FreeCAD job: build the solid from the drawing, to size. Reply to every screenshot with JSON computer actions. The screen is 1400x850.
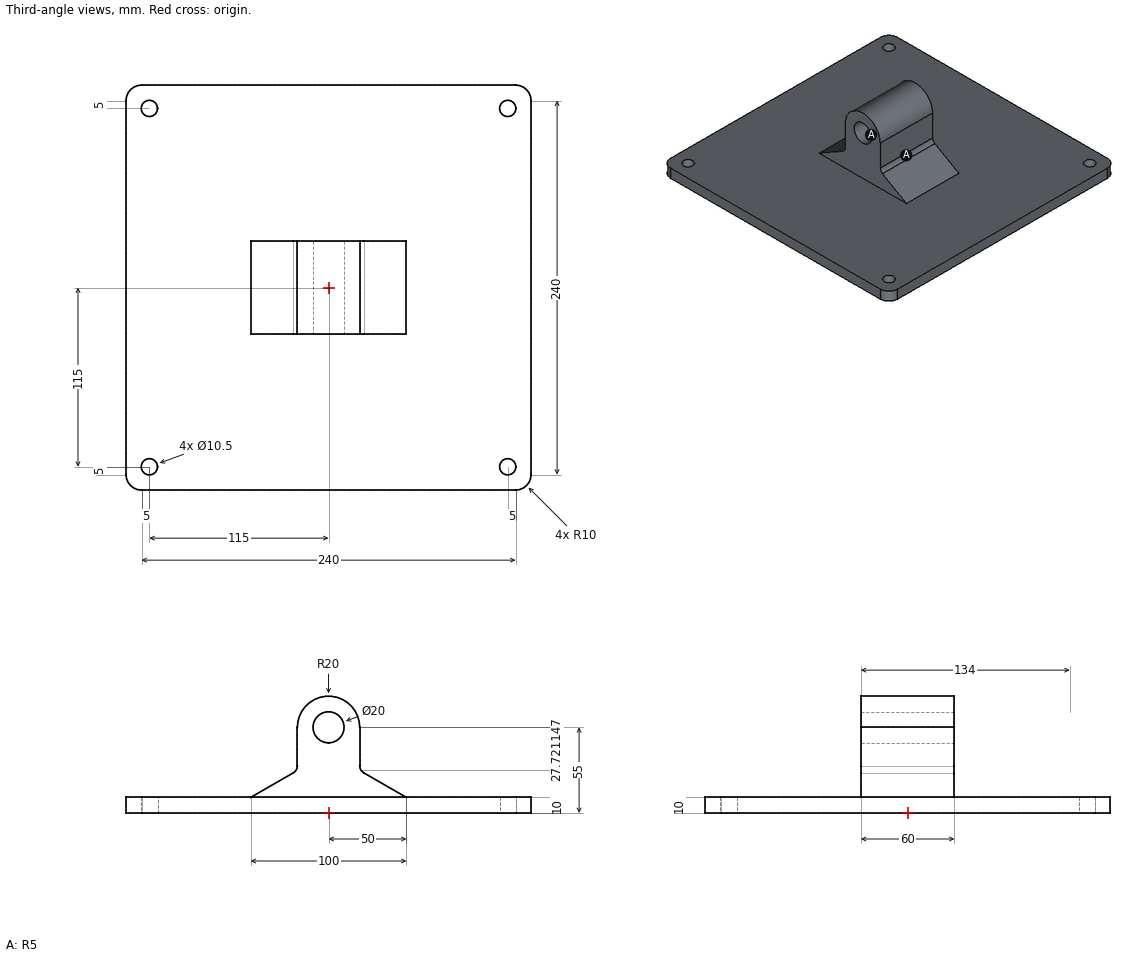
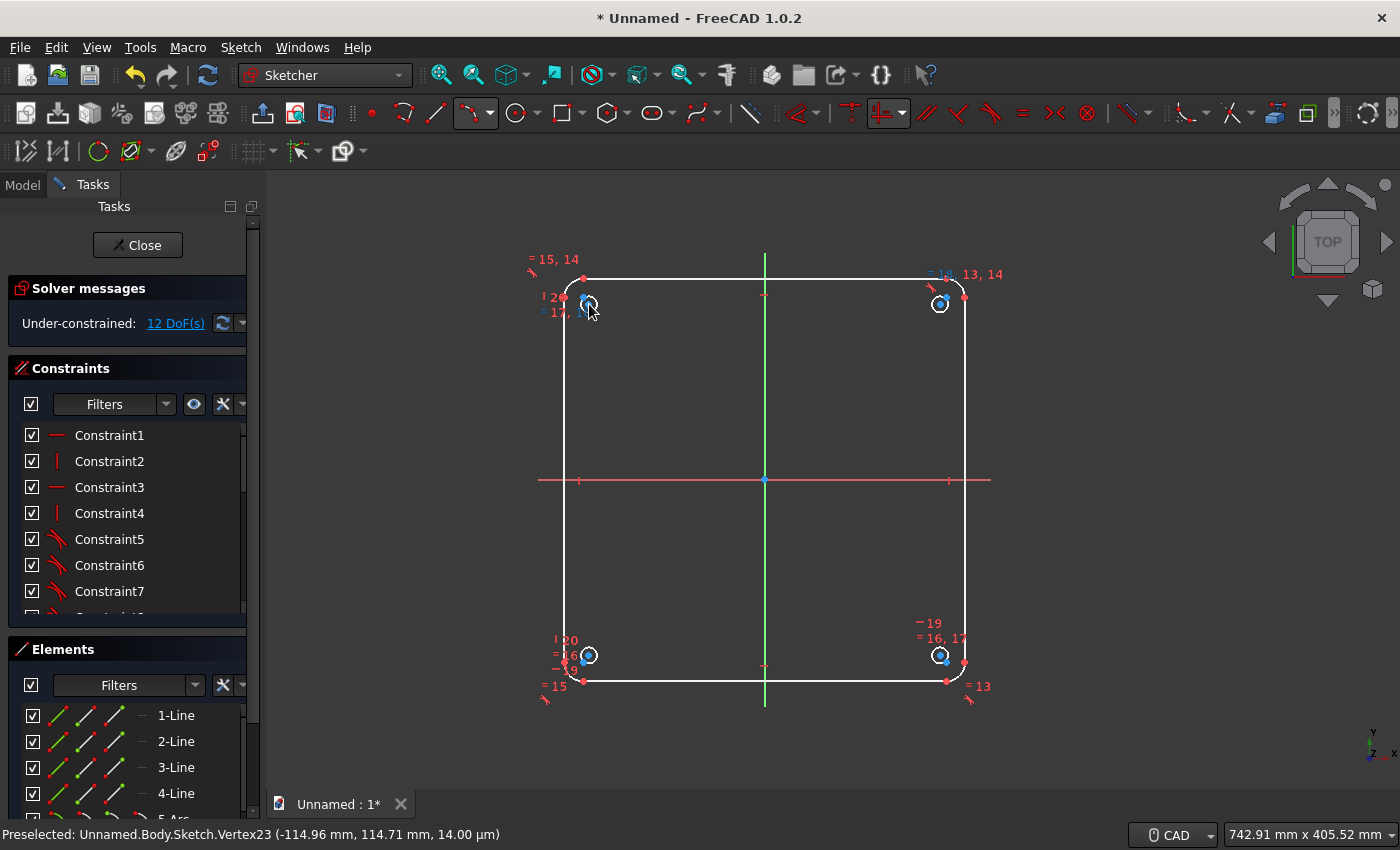
{"action": "scroll", "coordinate": [940, 655], "scroll_direction": "up", "scroll_amount": 2}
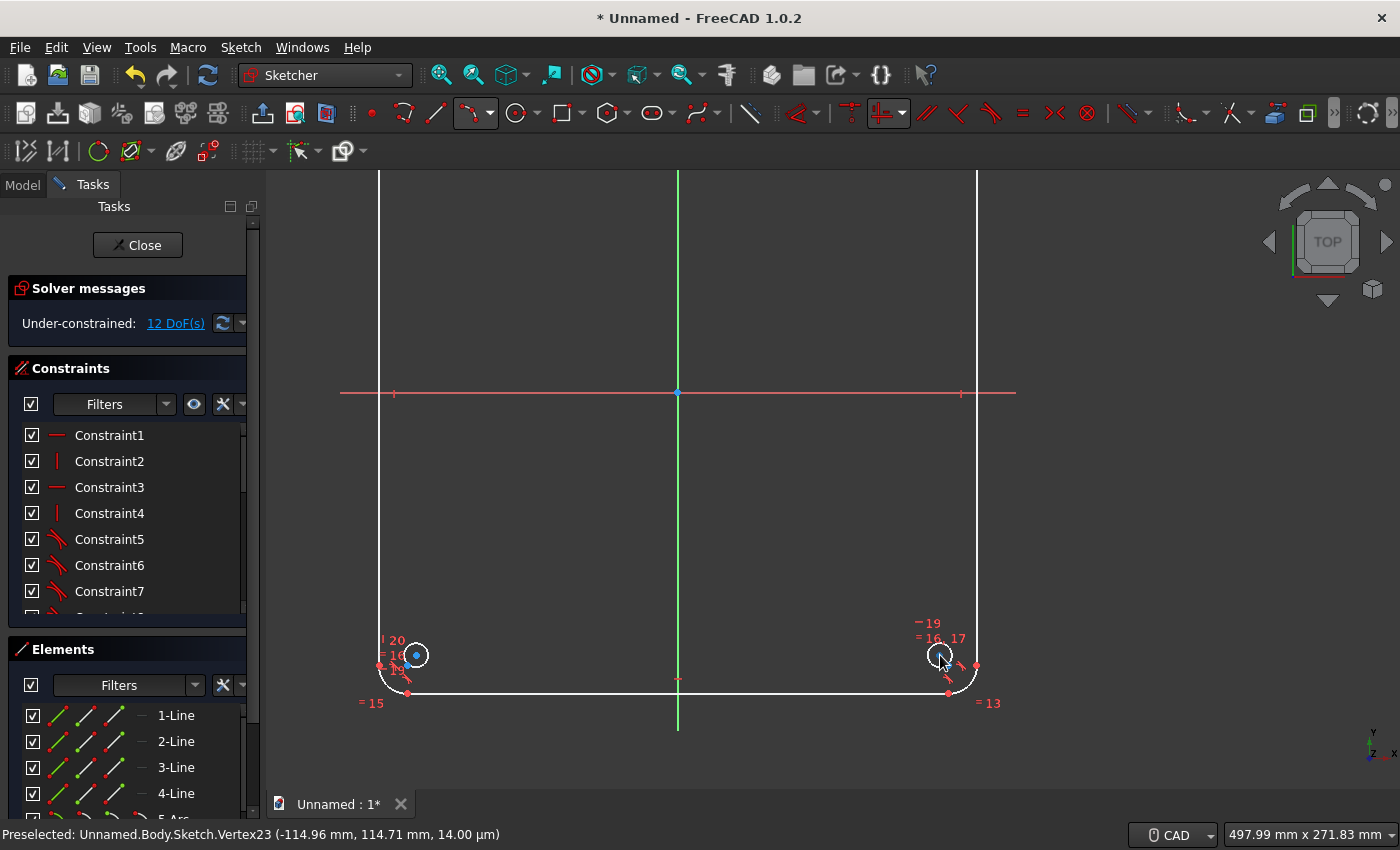
{"action": "left_click", "coordinate": [940, 655]}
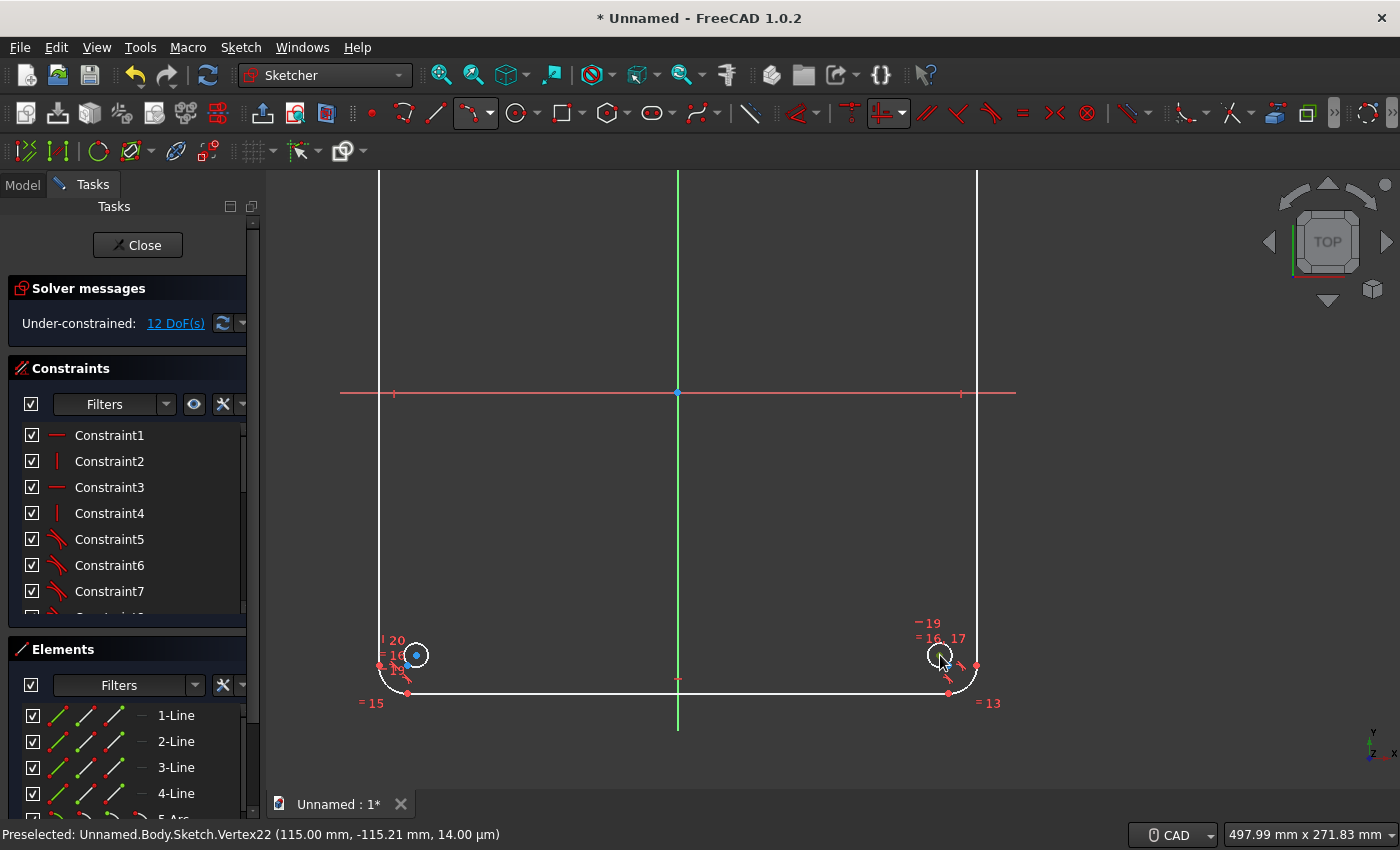
{"action": "scroll", "coordinate": [941, 656], "scroll_direction": "down", "scroll_amount": 2}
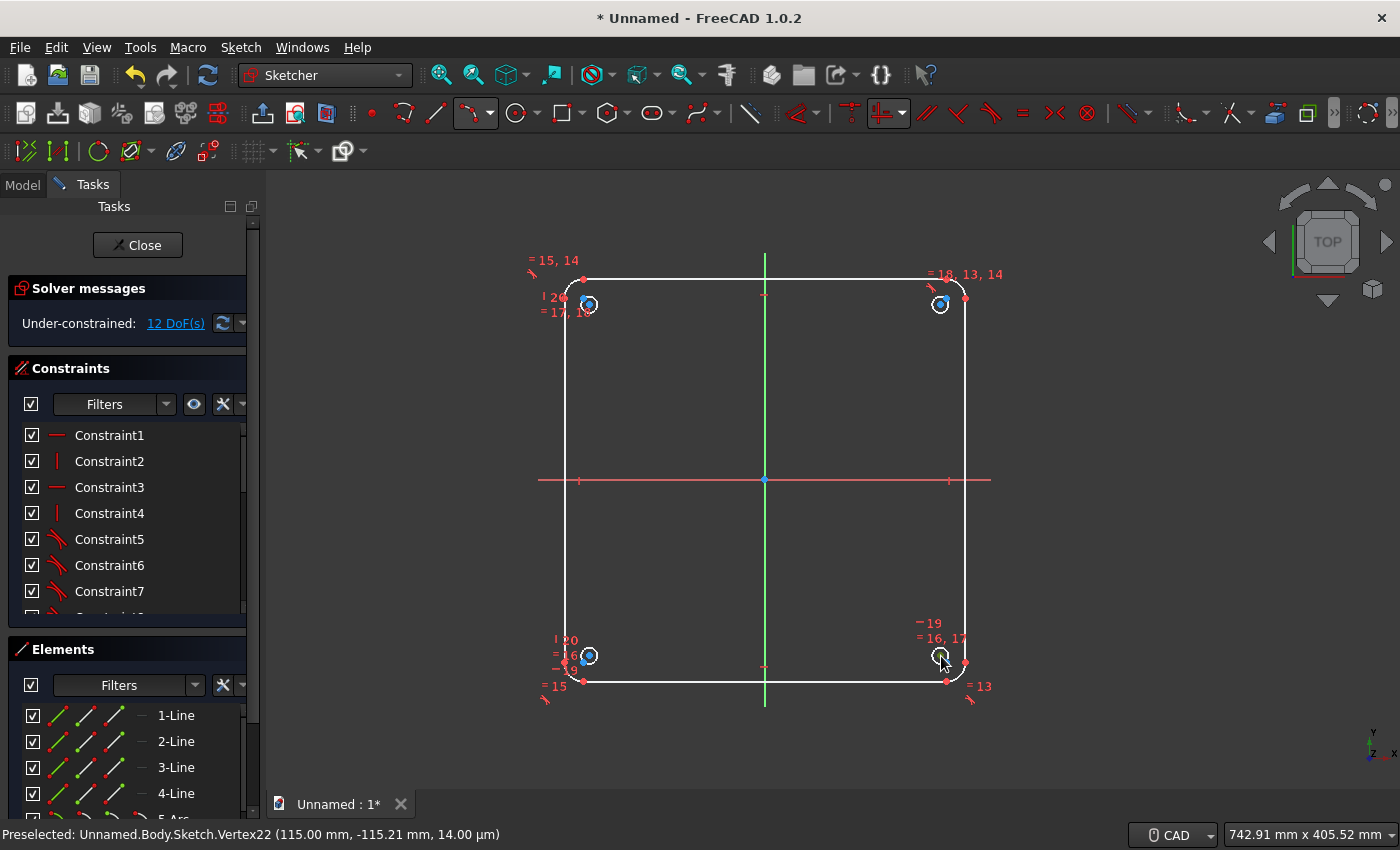
{"action": "scroll", "coordinate": [940, 305], "scroll_direction": "up", "scroll_amount": 2}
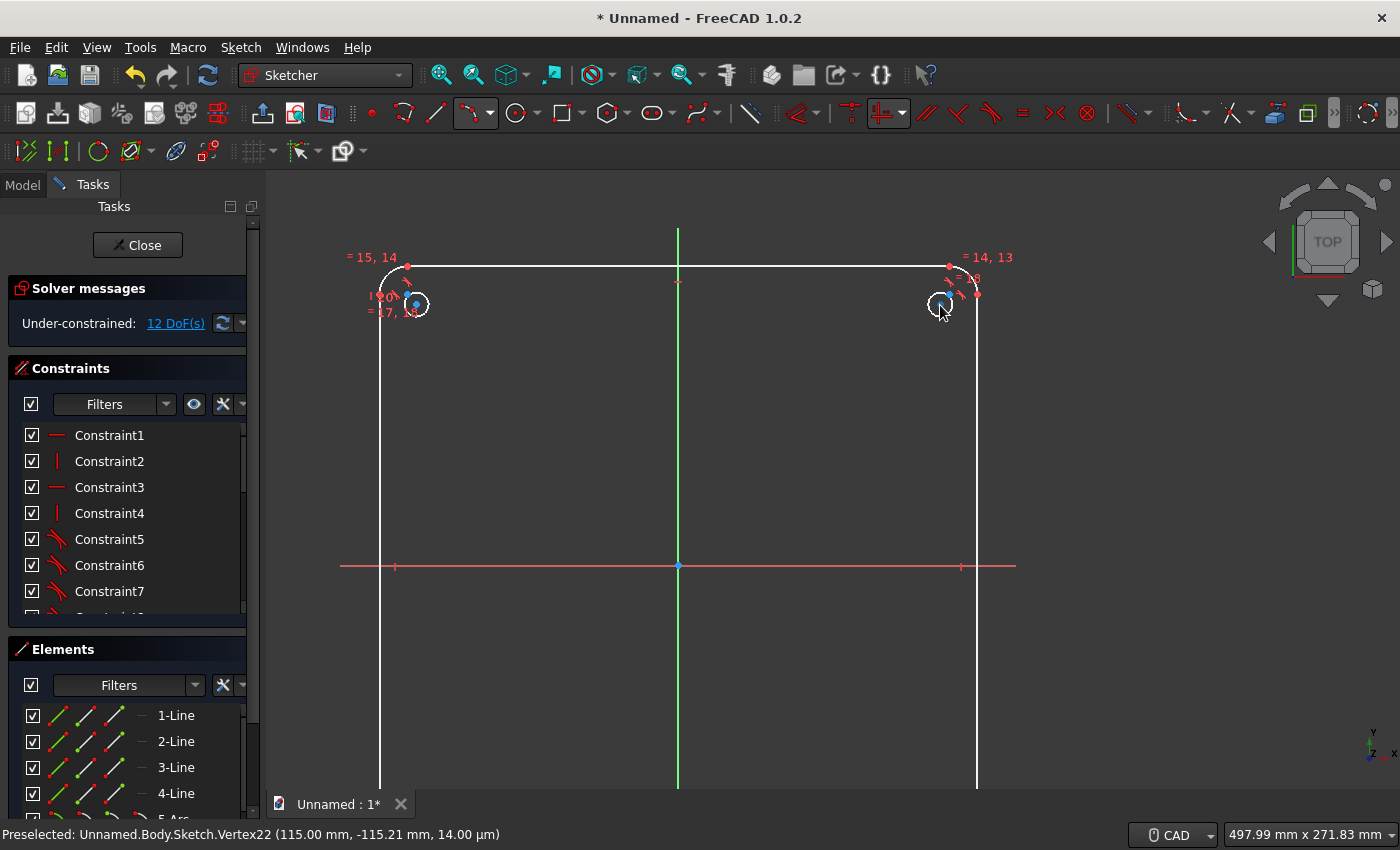
{"action": "left_click", "coordinate": [940, 305]}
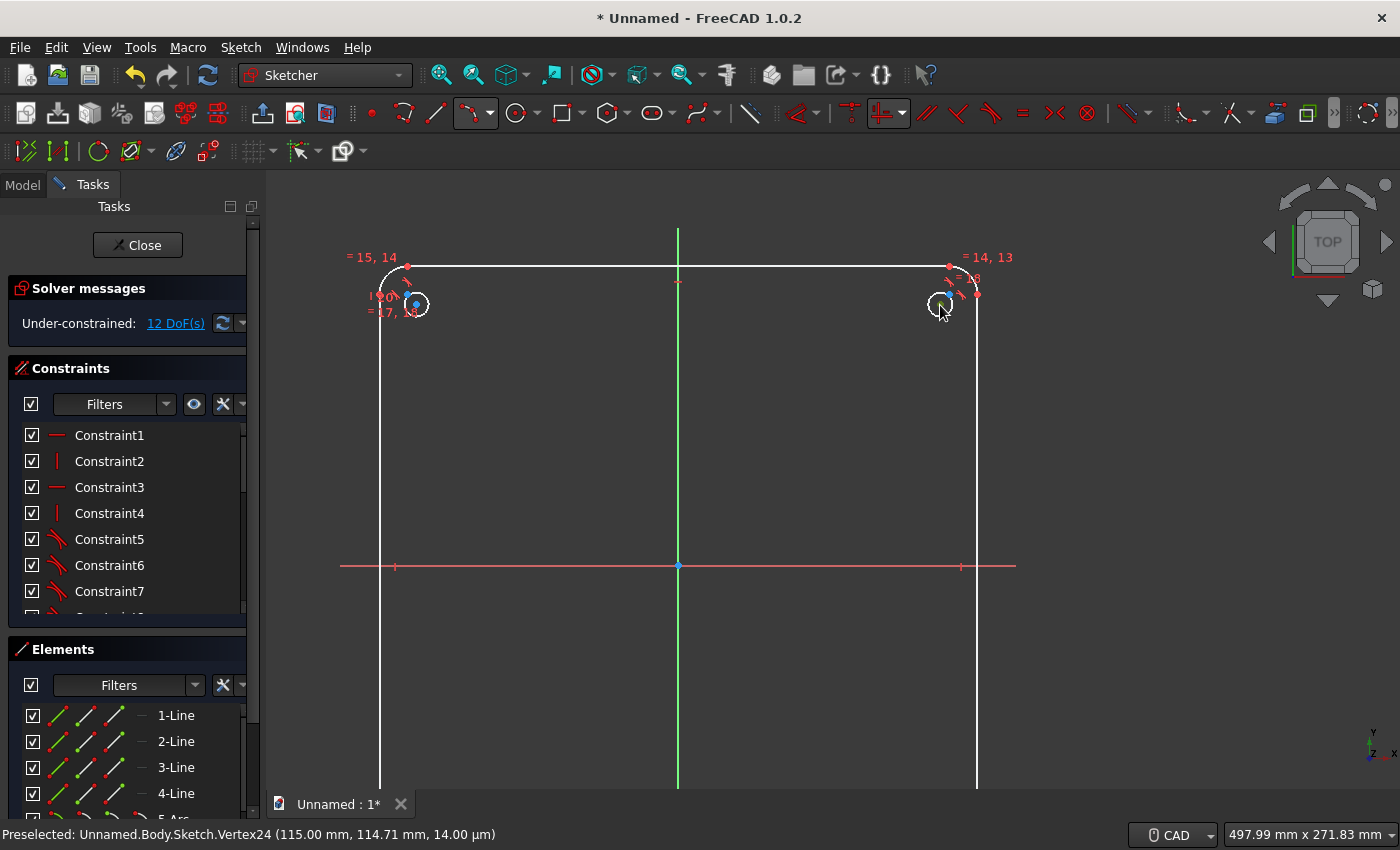
{"action": "key", "text": "v"}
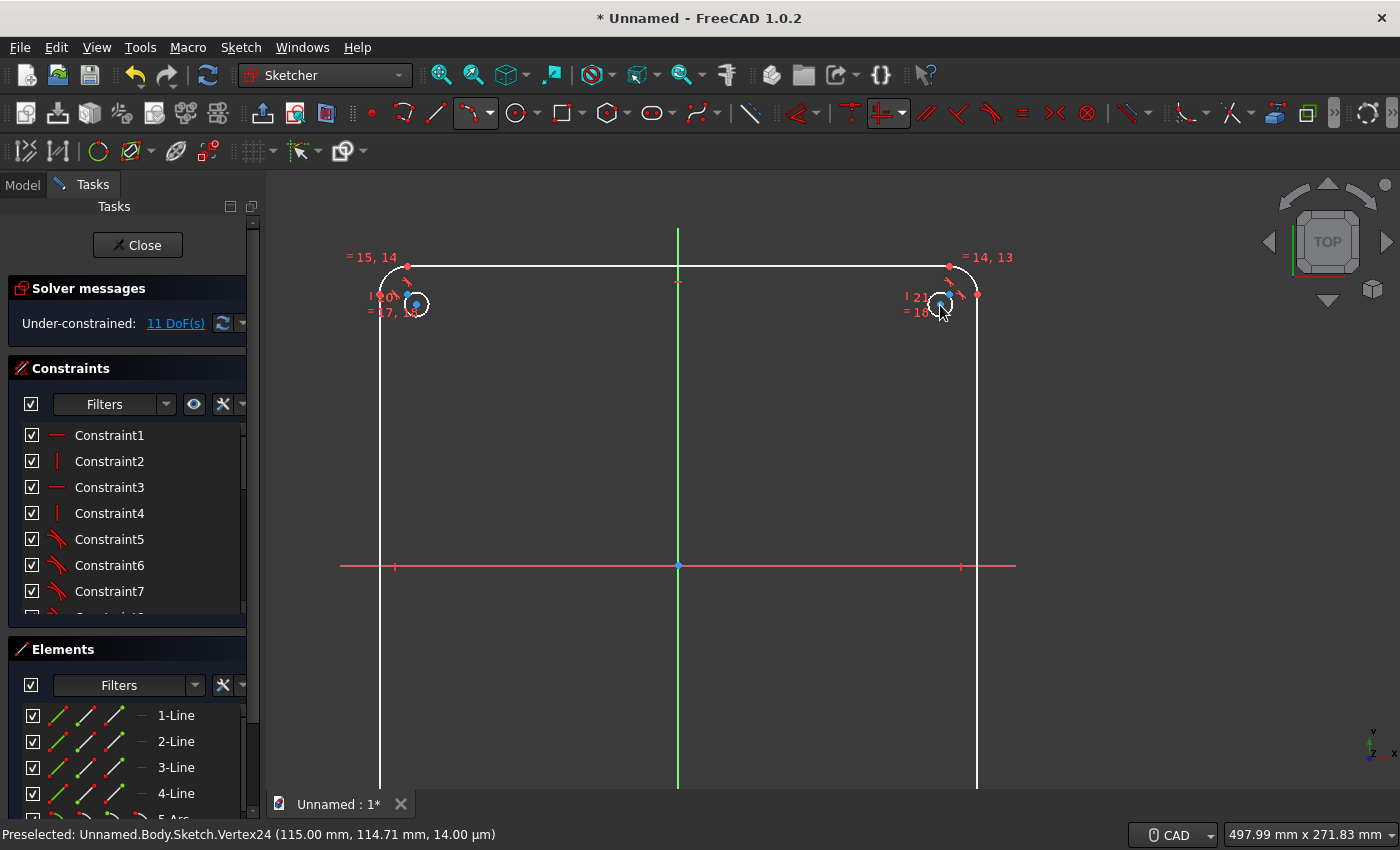
{"action": "left_click", "coordinate": [419, 307]}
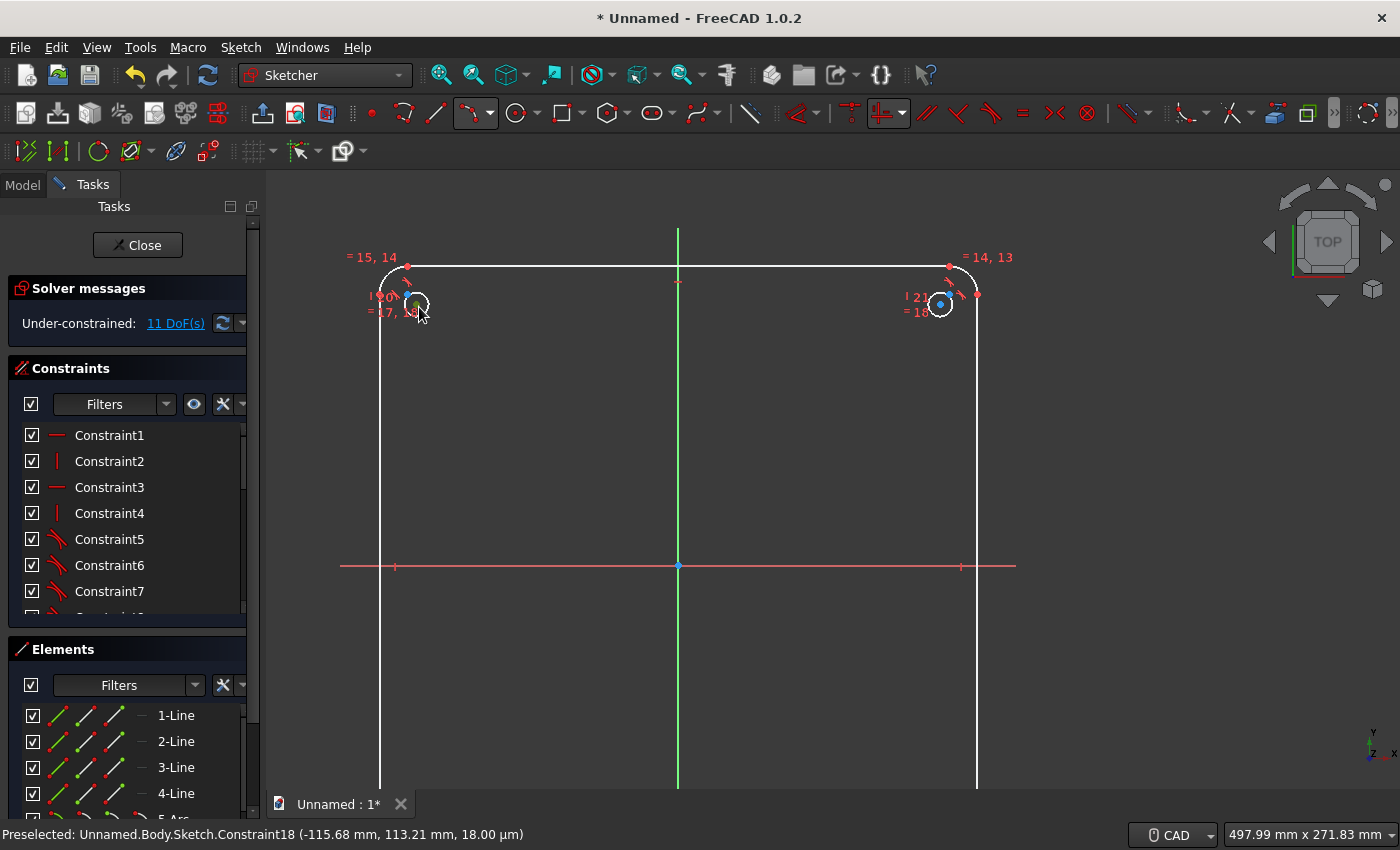
{"action": "left_click", "coordinate": [940, 305]}